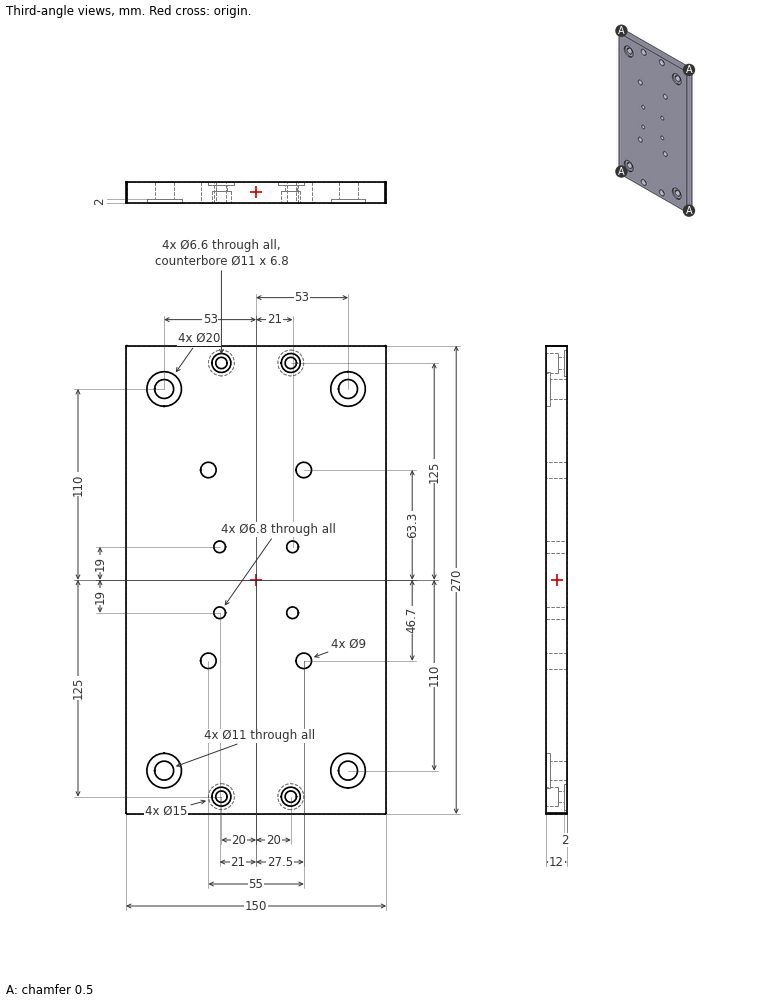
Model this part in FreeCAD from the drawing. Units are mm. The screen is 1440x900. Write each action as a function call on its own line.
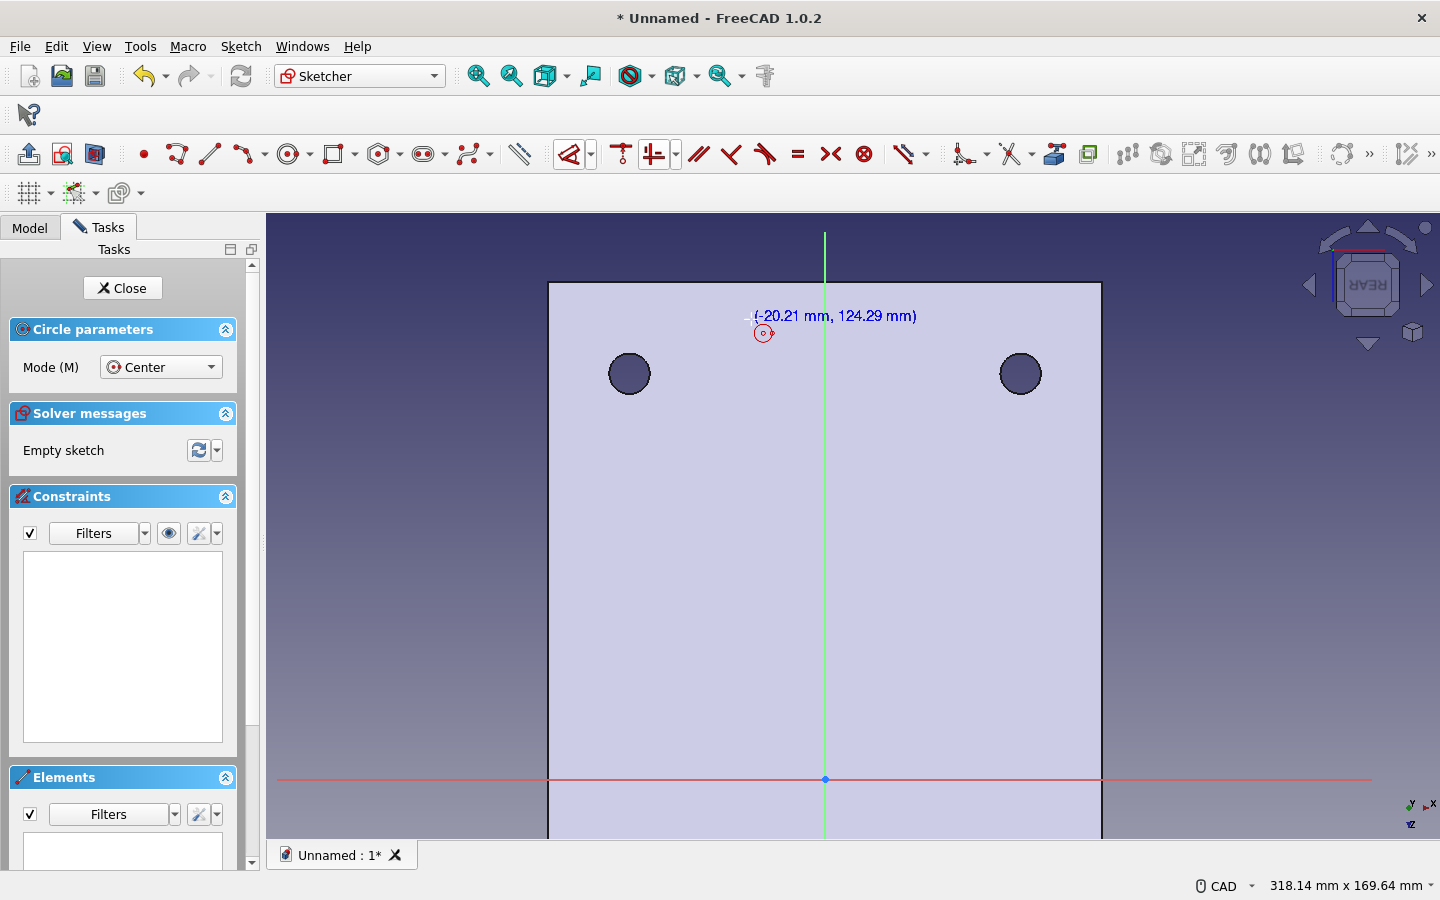
click(751, 318)
click(771, 299)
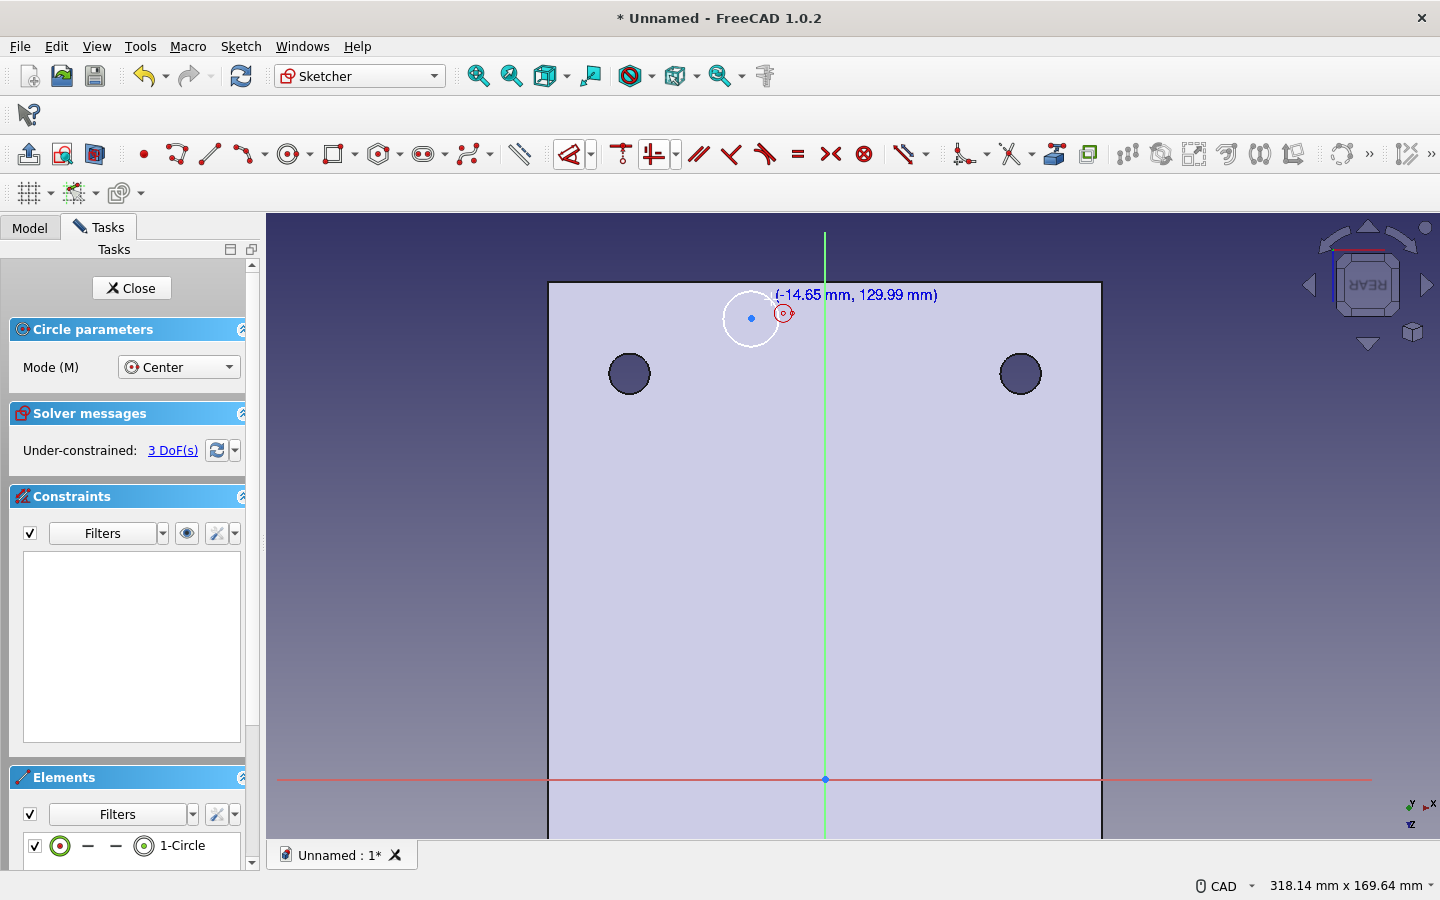
click(899, 318)
click(918, 299)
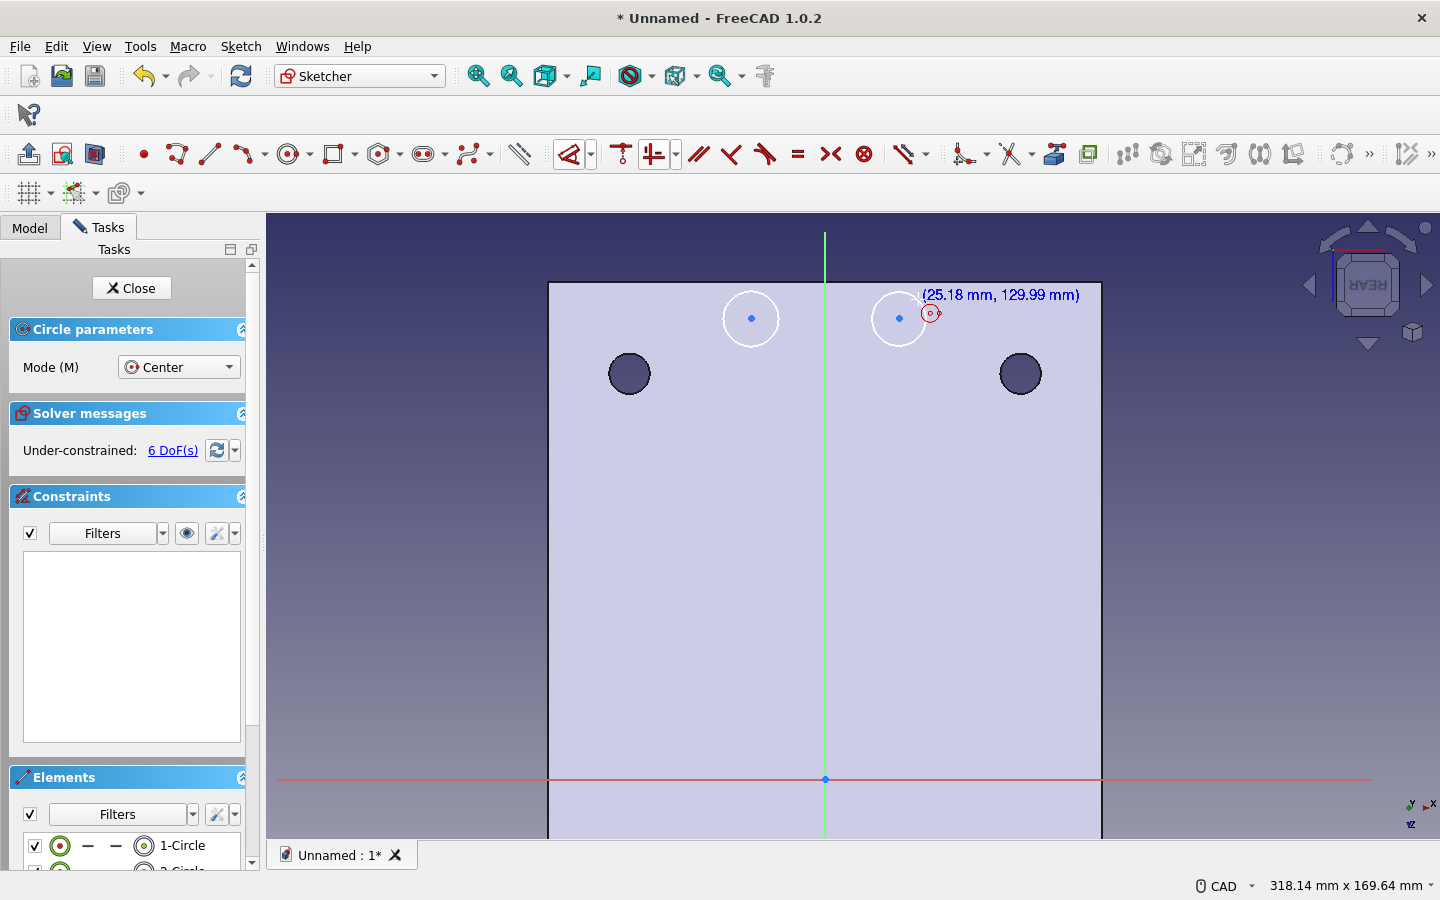
scroll(751, 319, down, 4)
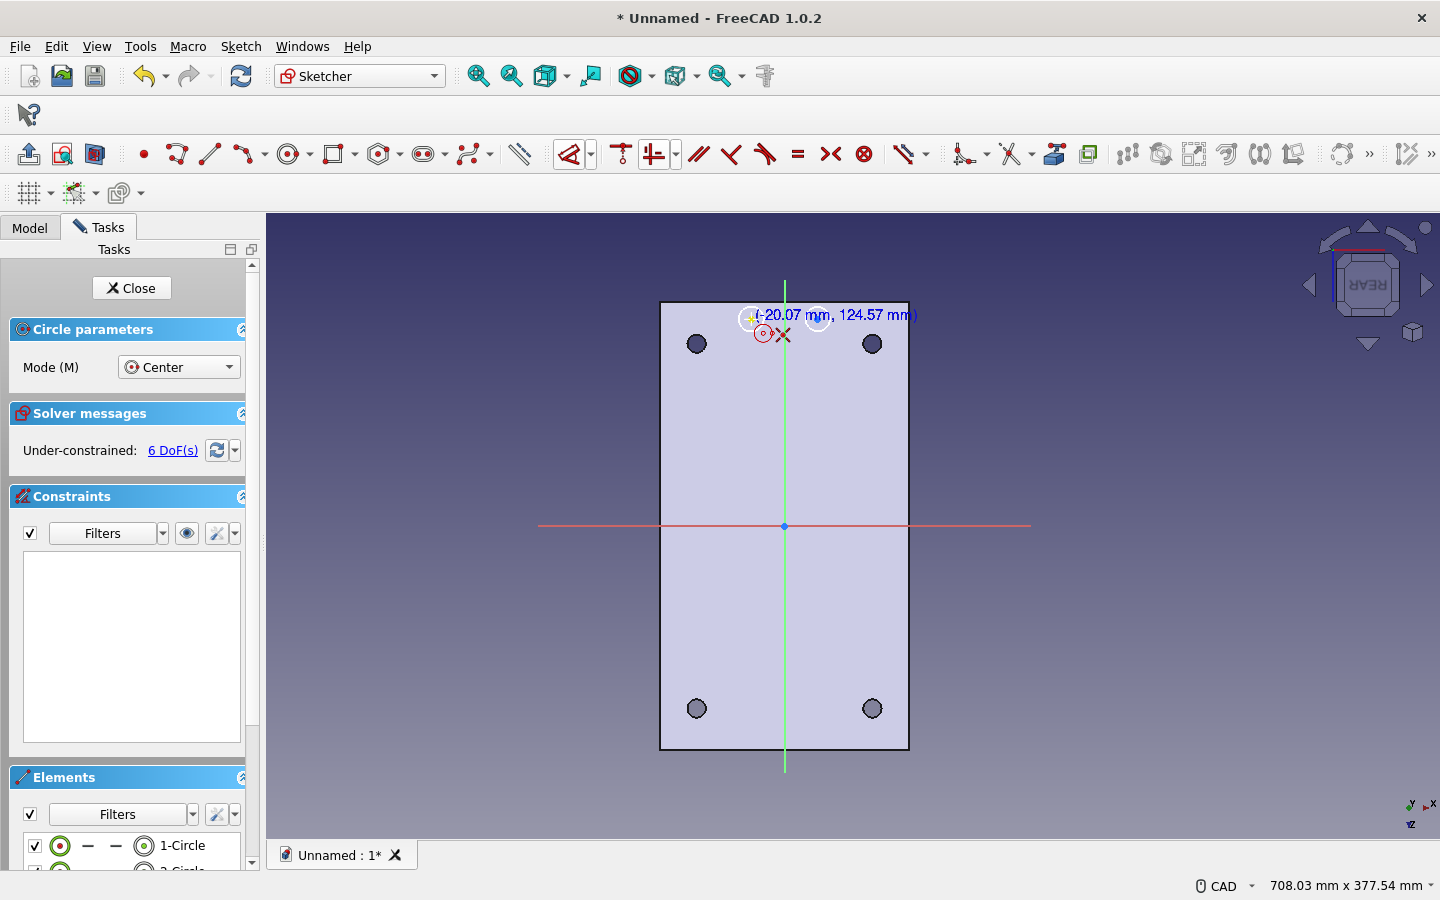
scroll(818, 733, up, 4)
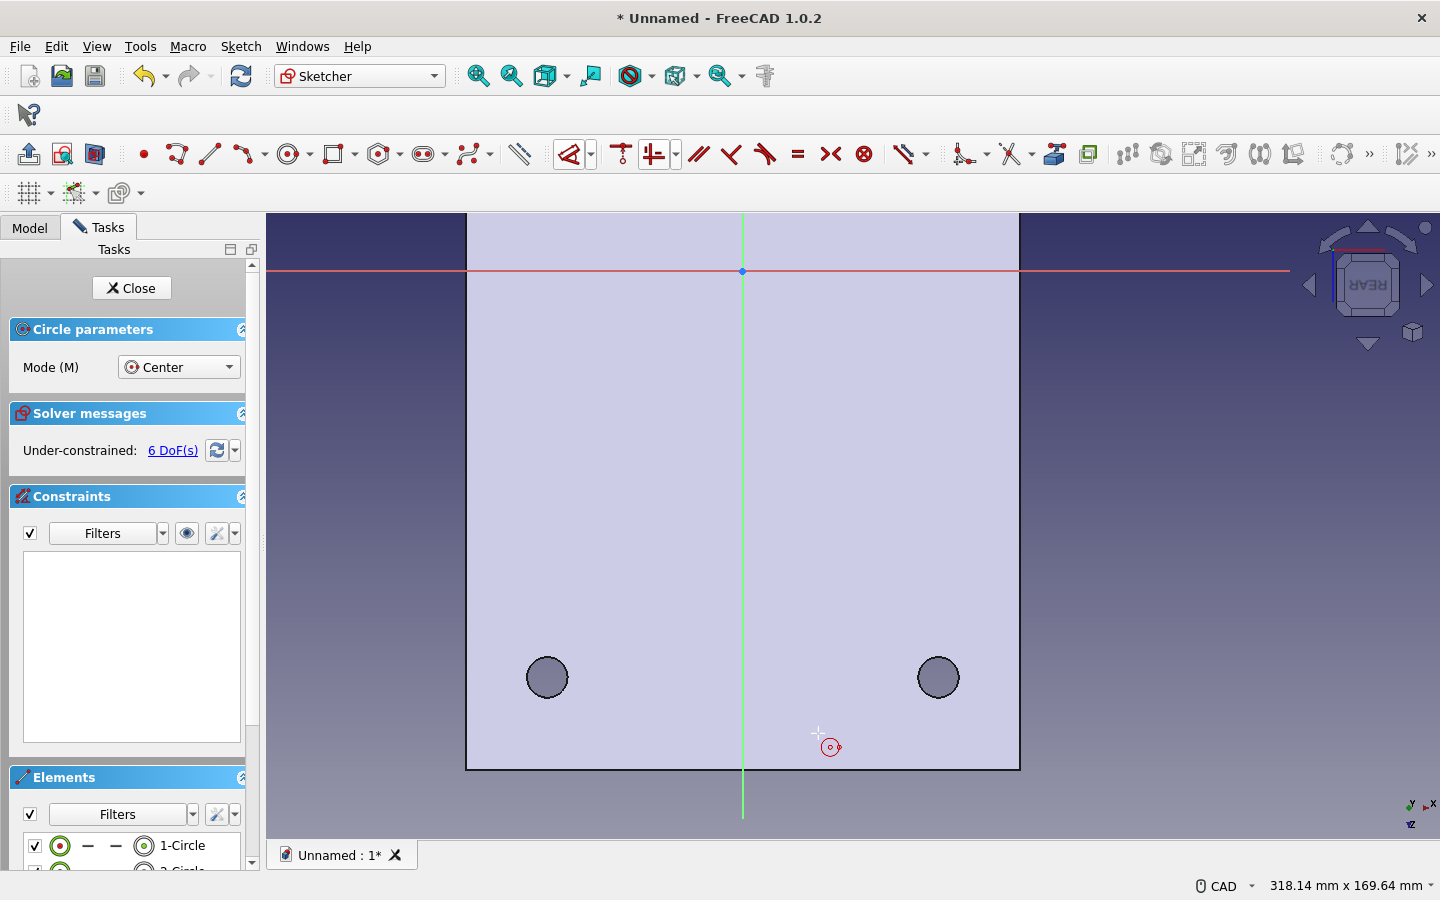
click(817, 733)
click(836, 713)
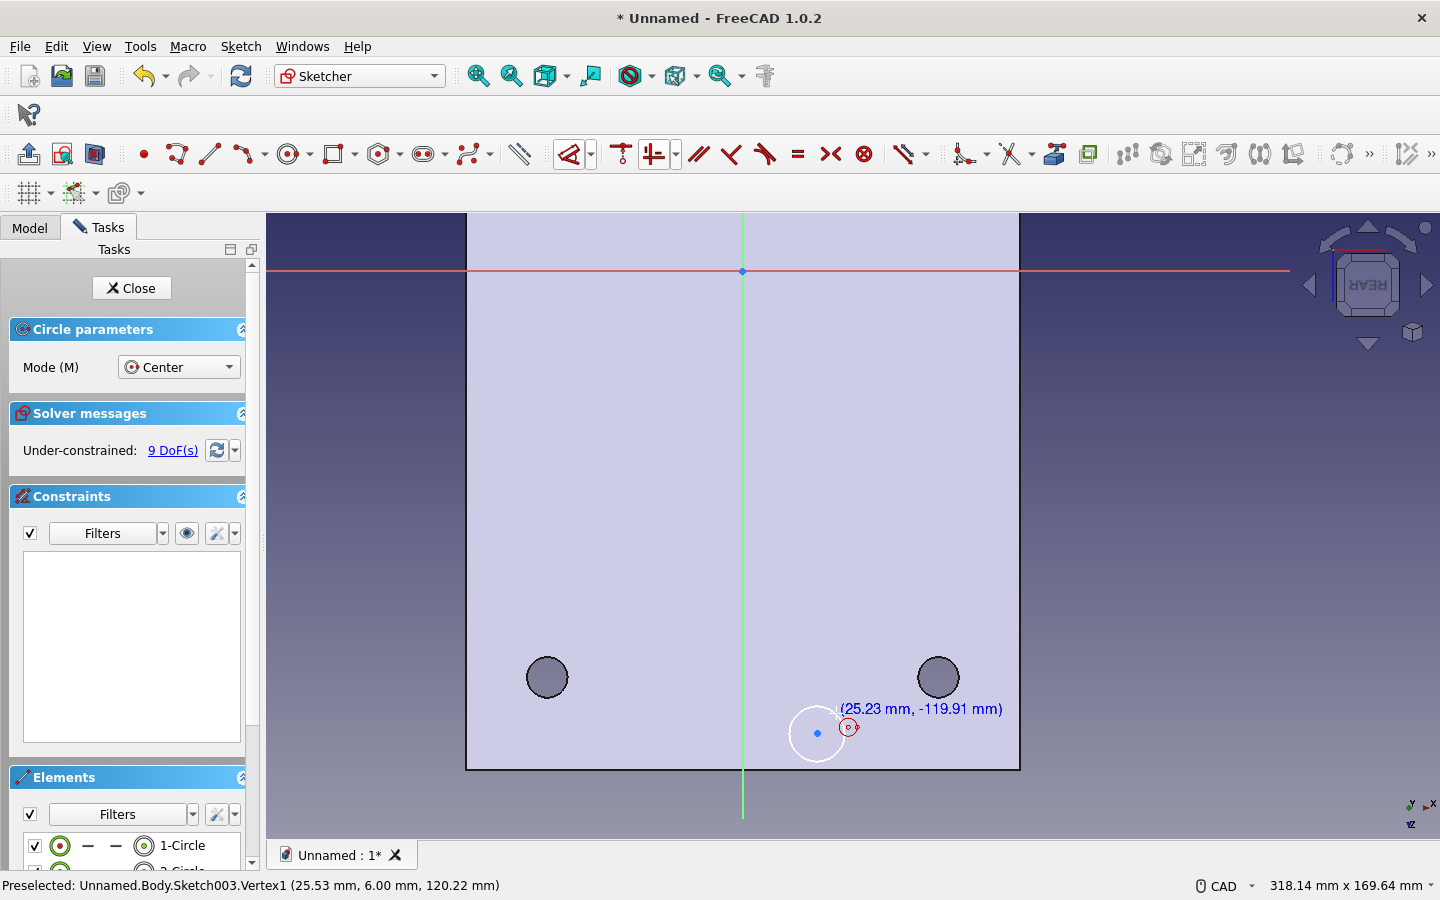
click(669, 733)
click(689, 713)
key(Escape)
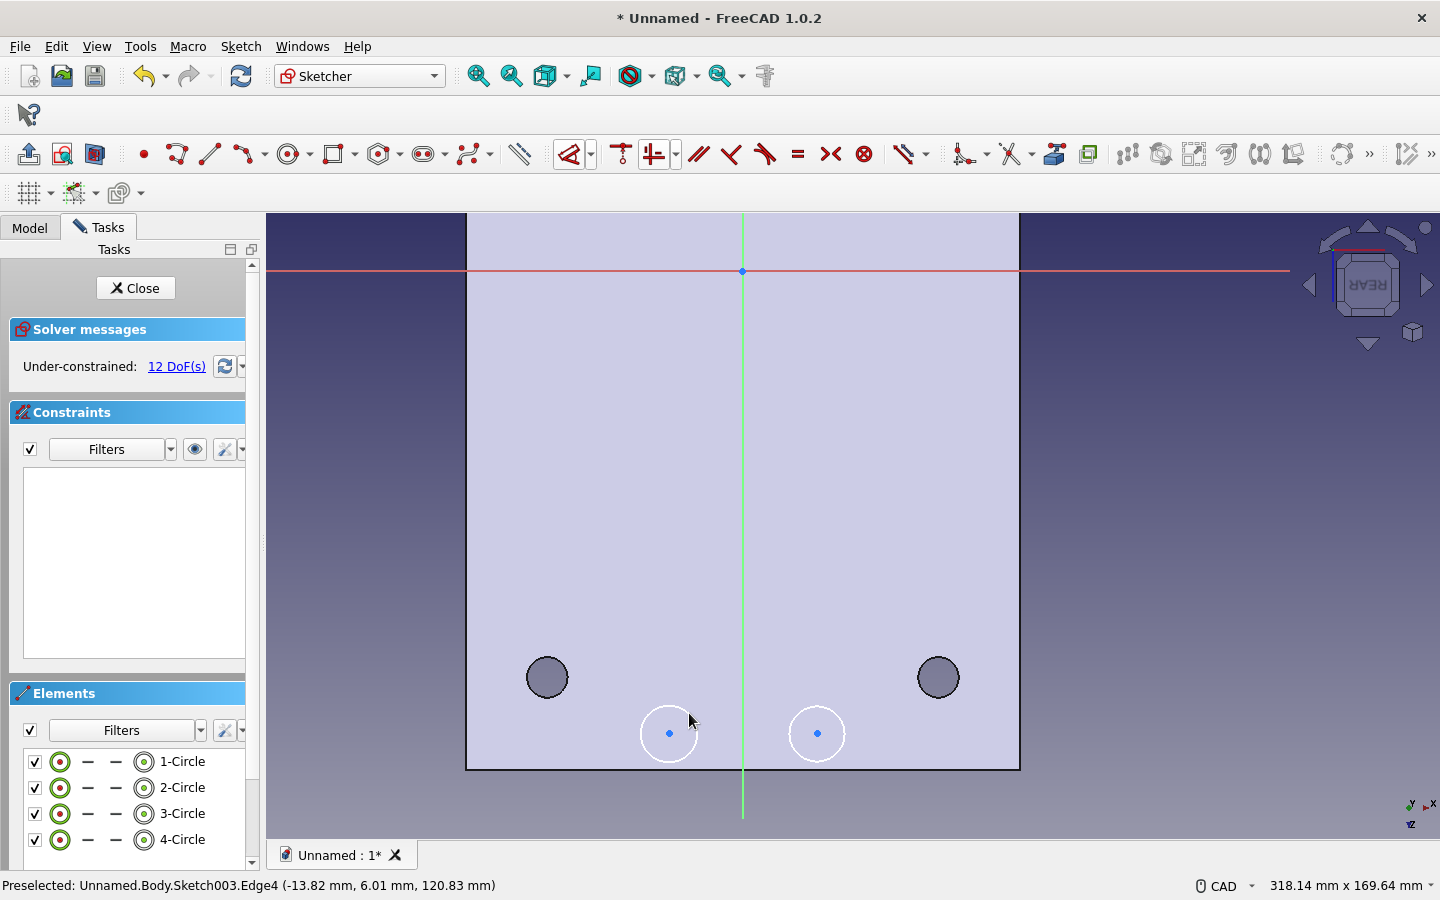
scroll(818, 734, down, 4)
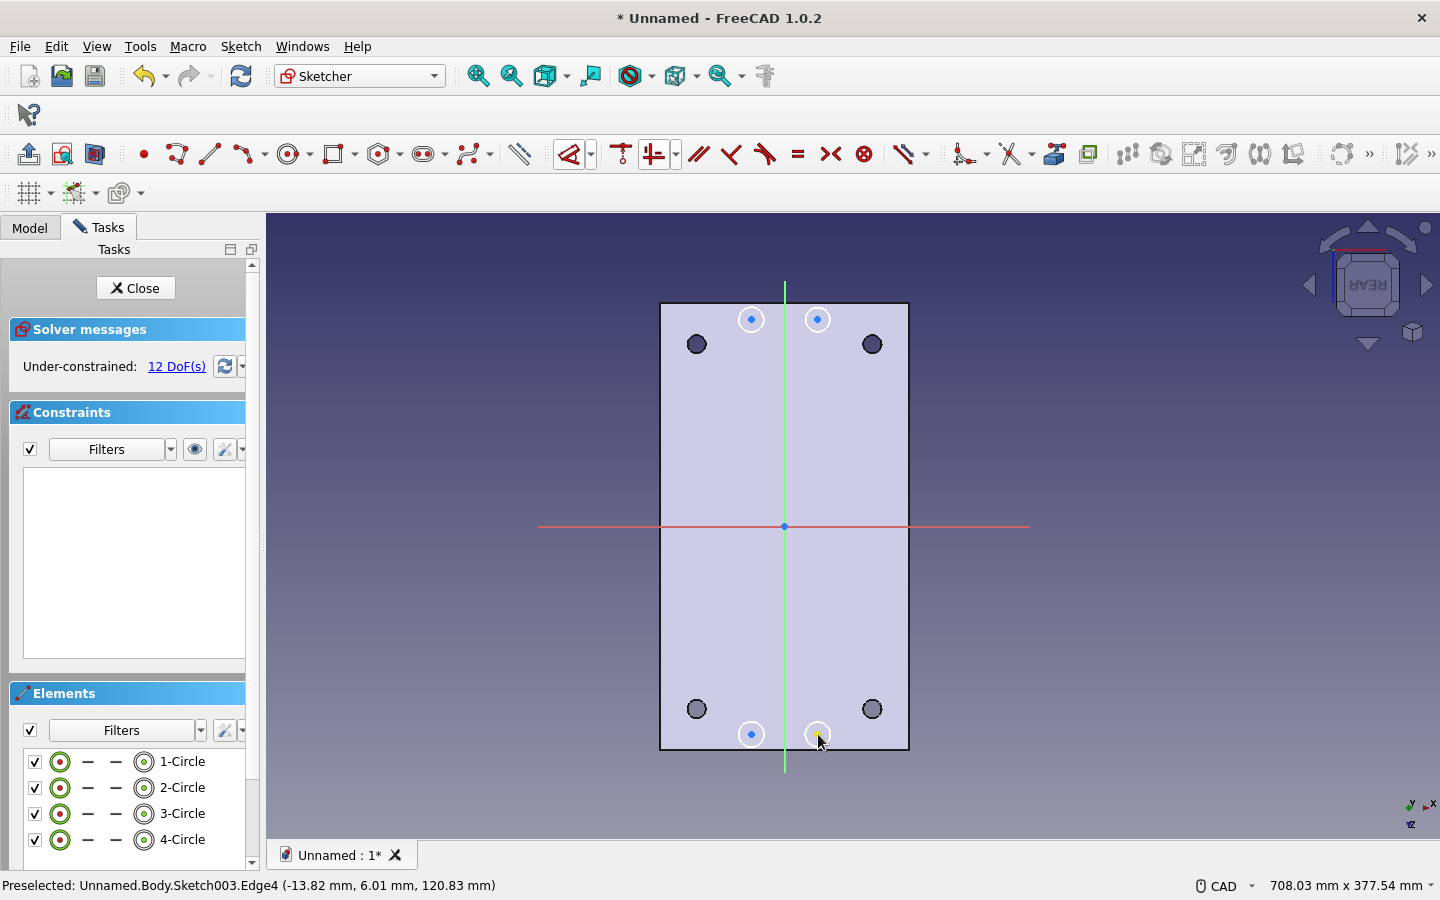
click(760, 311)